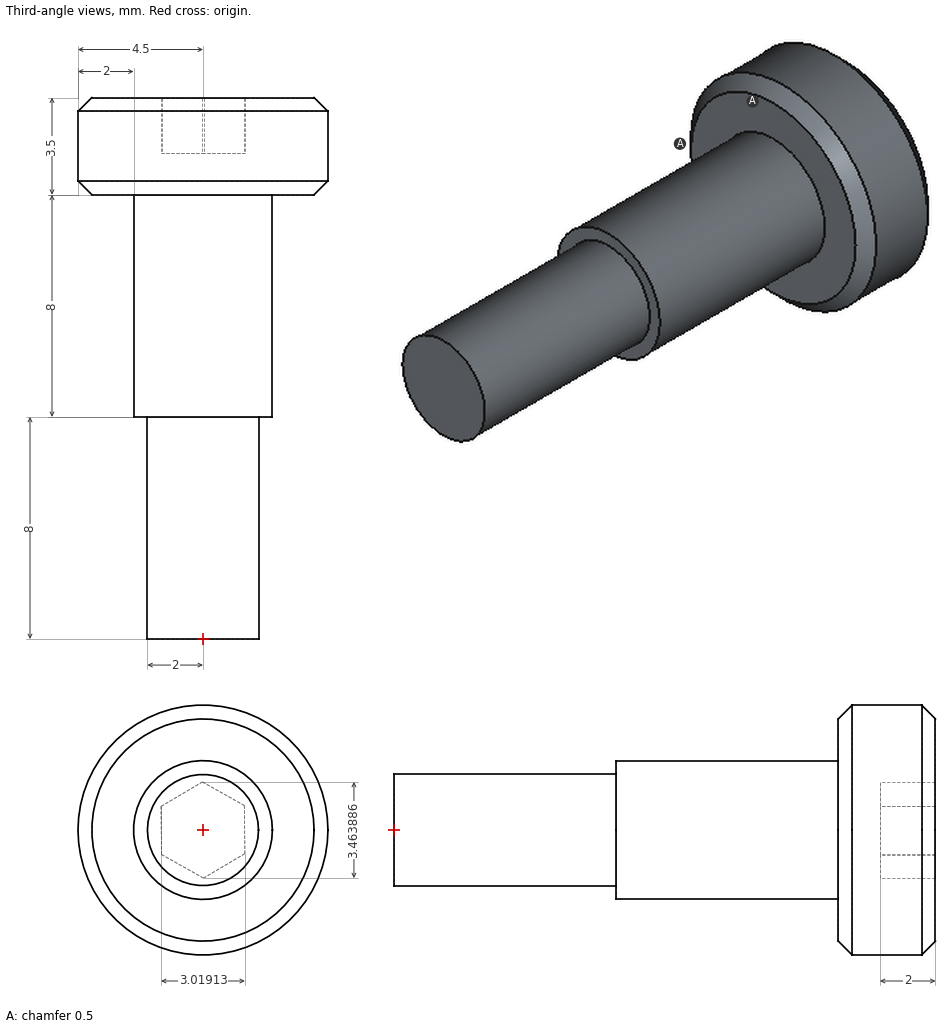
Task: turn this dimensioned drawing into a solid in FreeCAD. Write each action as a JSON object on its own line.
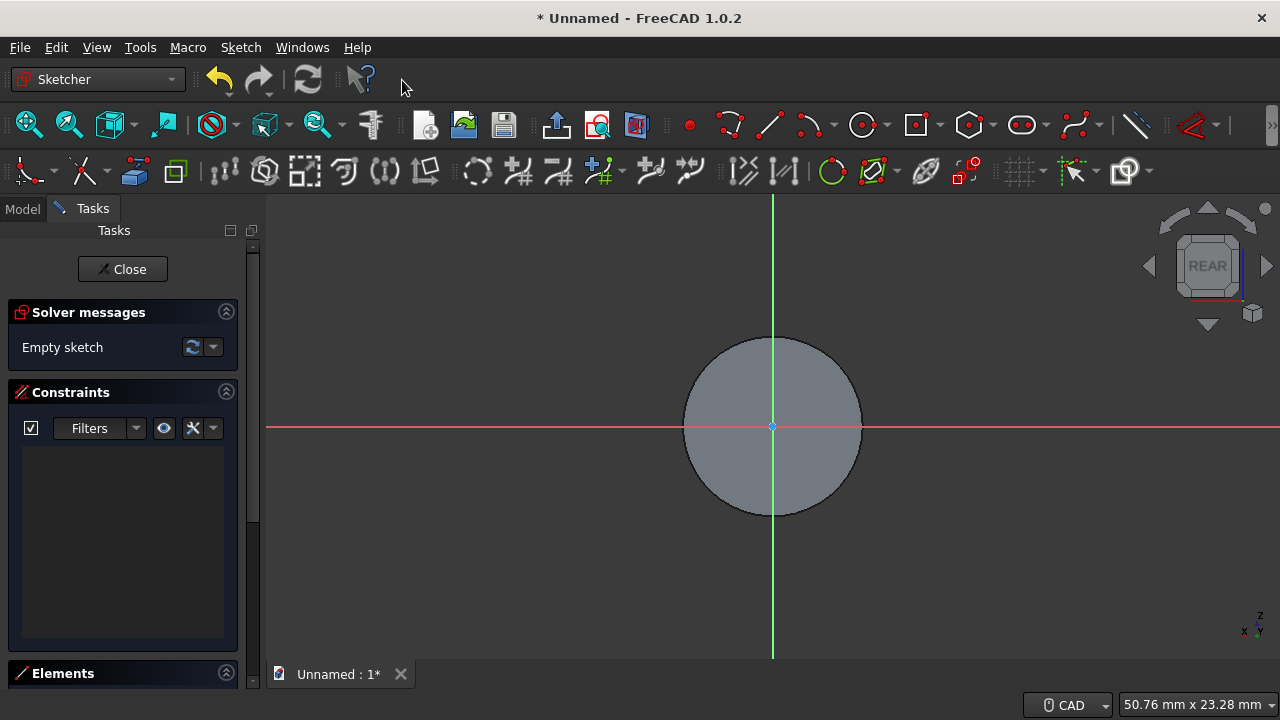
{"action": "scroll", "coordinate": [795, 426], "scroll_direction": "up", "scroll_amount": 7}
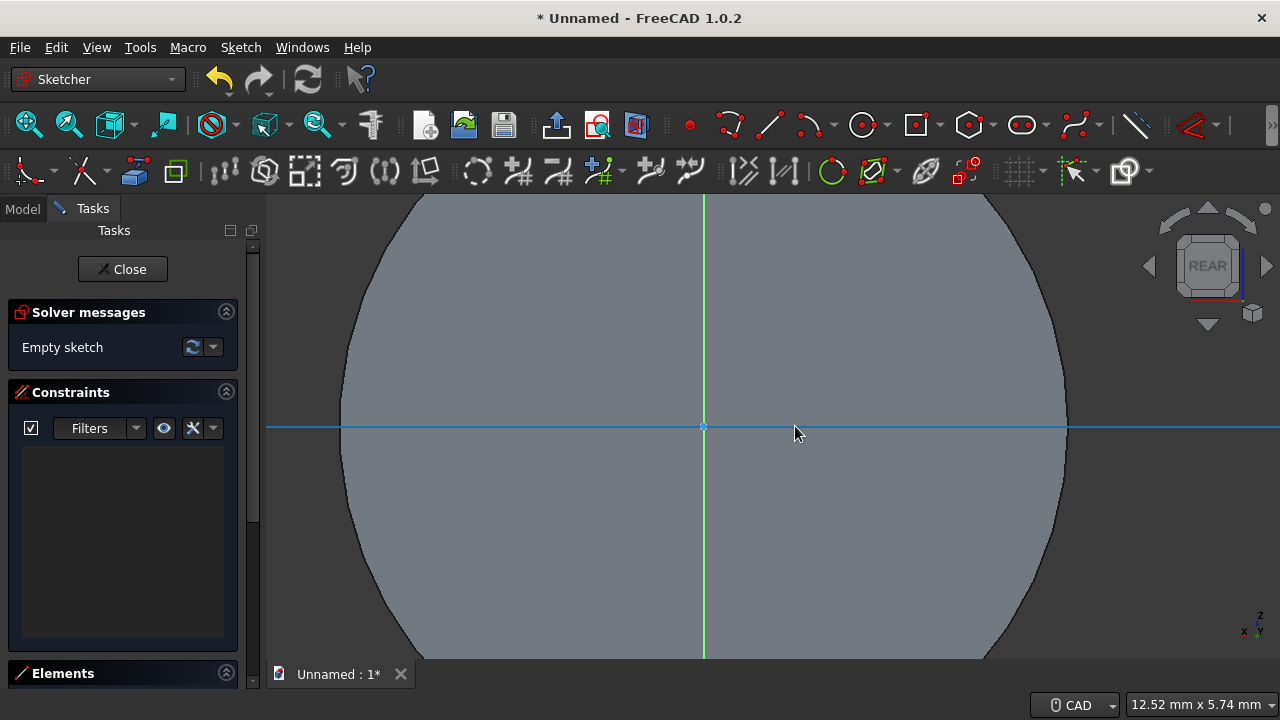
{"action": "left_click", "coordinate": [970, 126]}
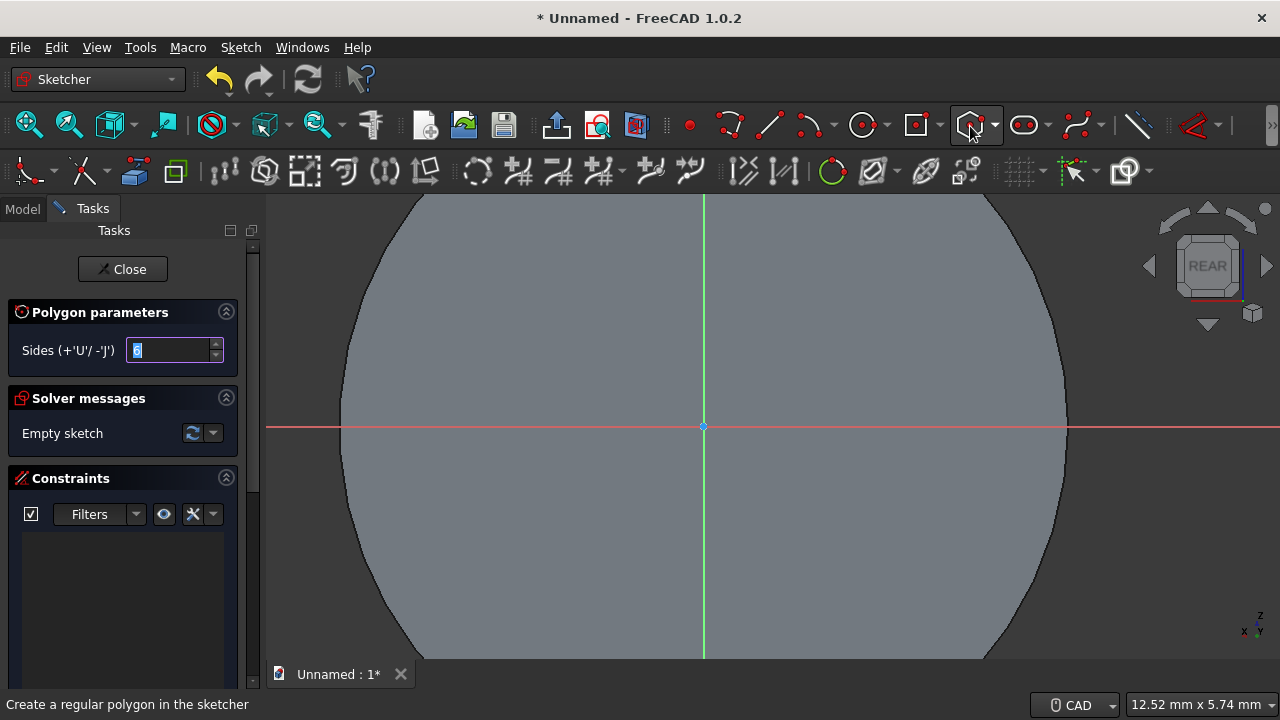
{"action": "left_click", "coordinate": [704, 426]}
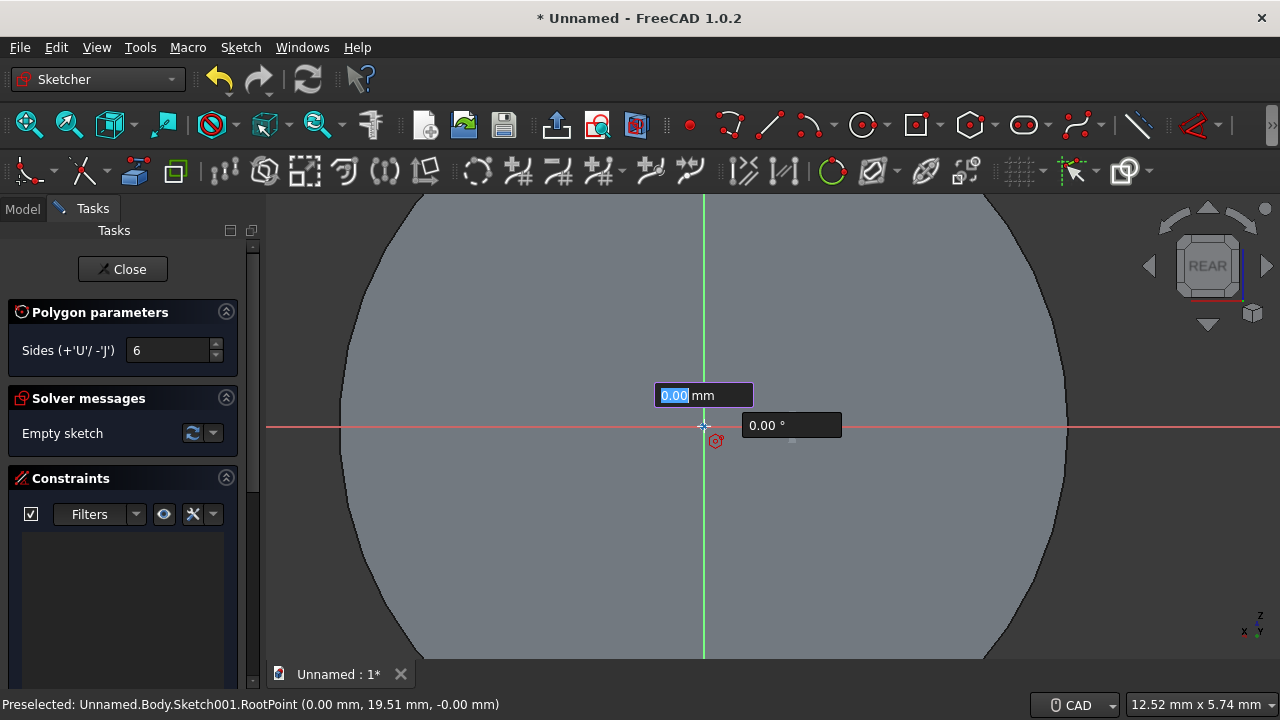
{"action": "left_click", "coordinate": [824, 498]}
{"action": "right_click", "coordinate": [824, 498]}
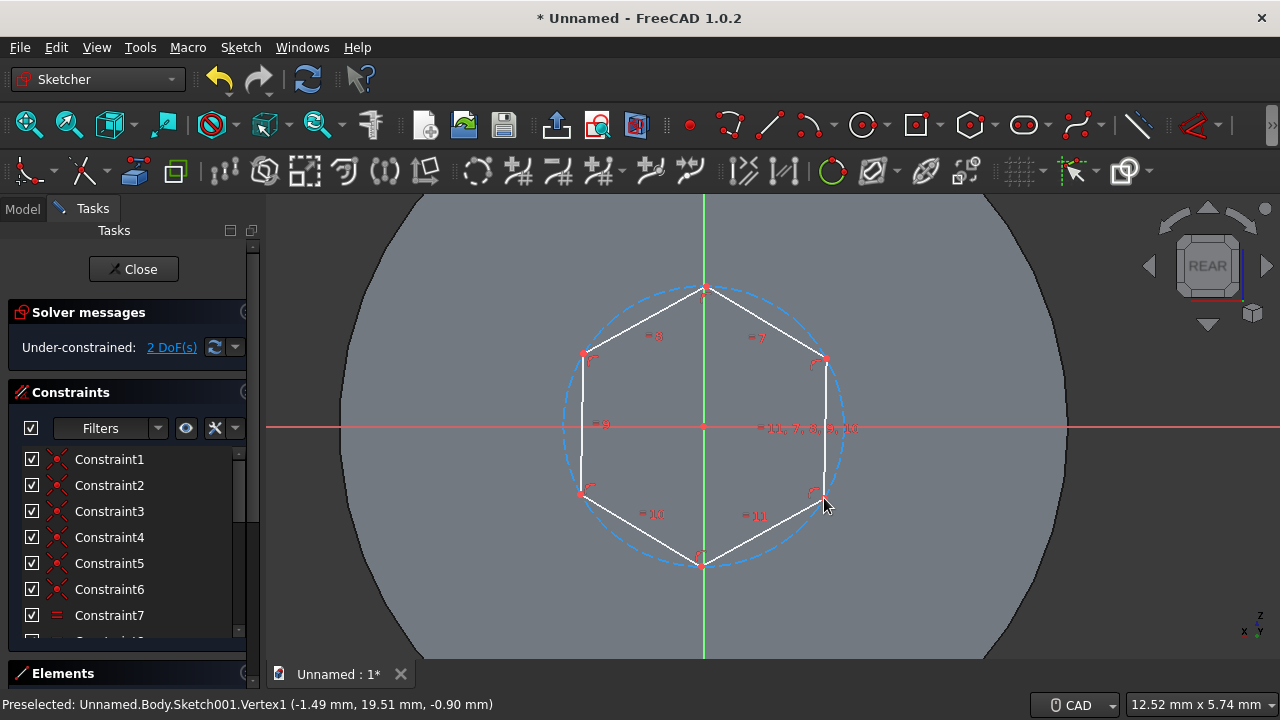
{"action": "key", "text": "d"}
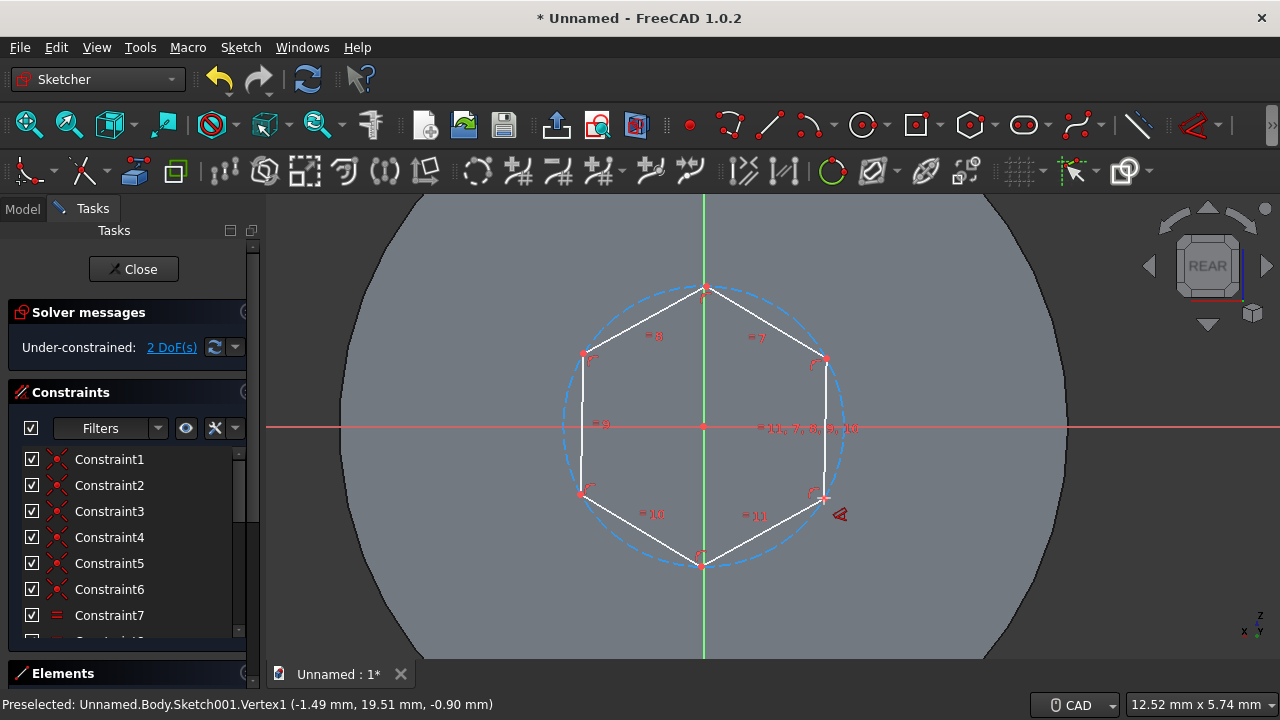
{"action": "left_click", "coordinate": [581, 494]}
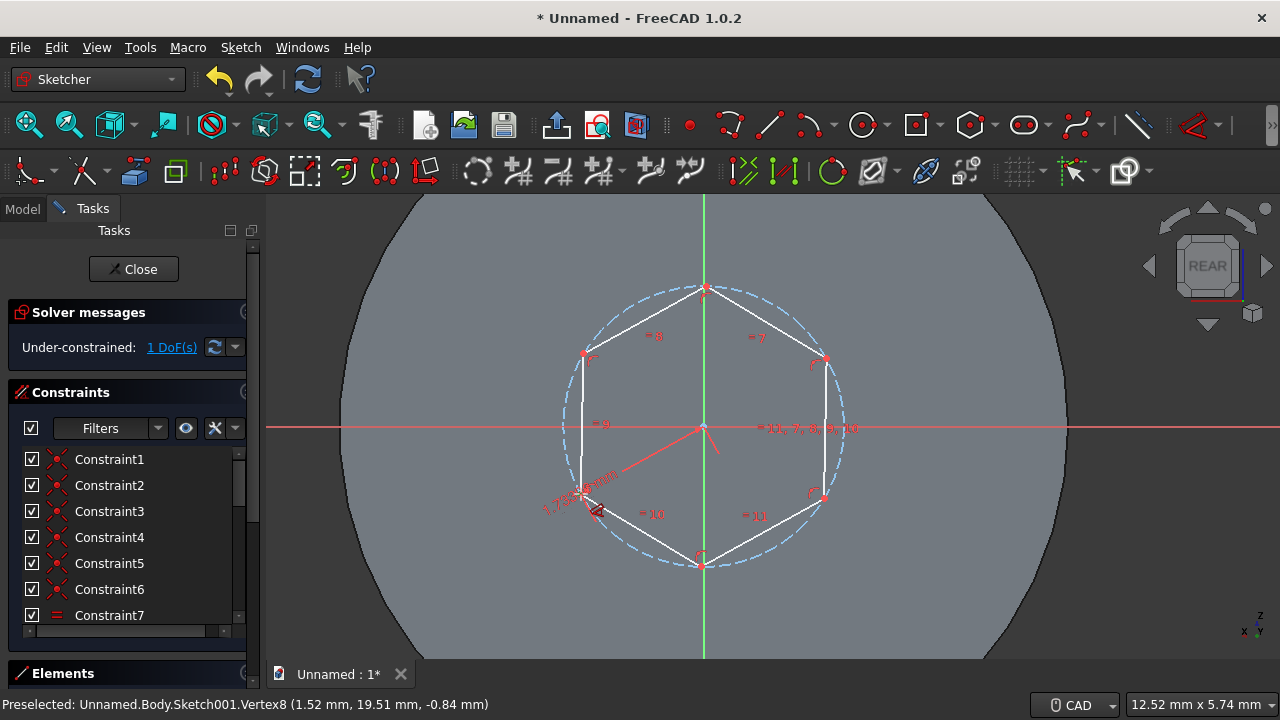
{"action": "left_click", "coordinate": [827, 359]}
{"action": "left_click", "coordinate": [647, 576]}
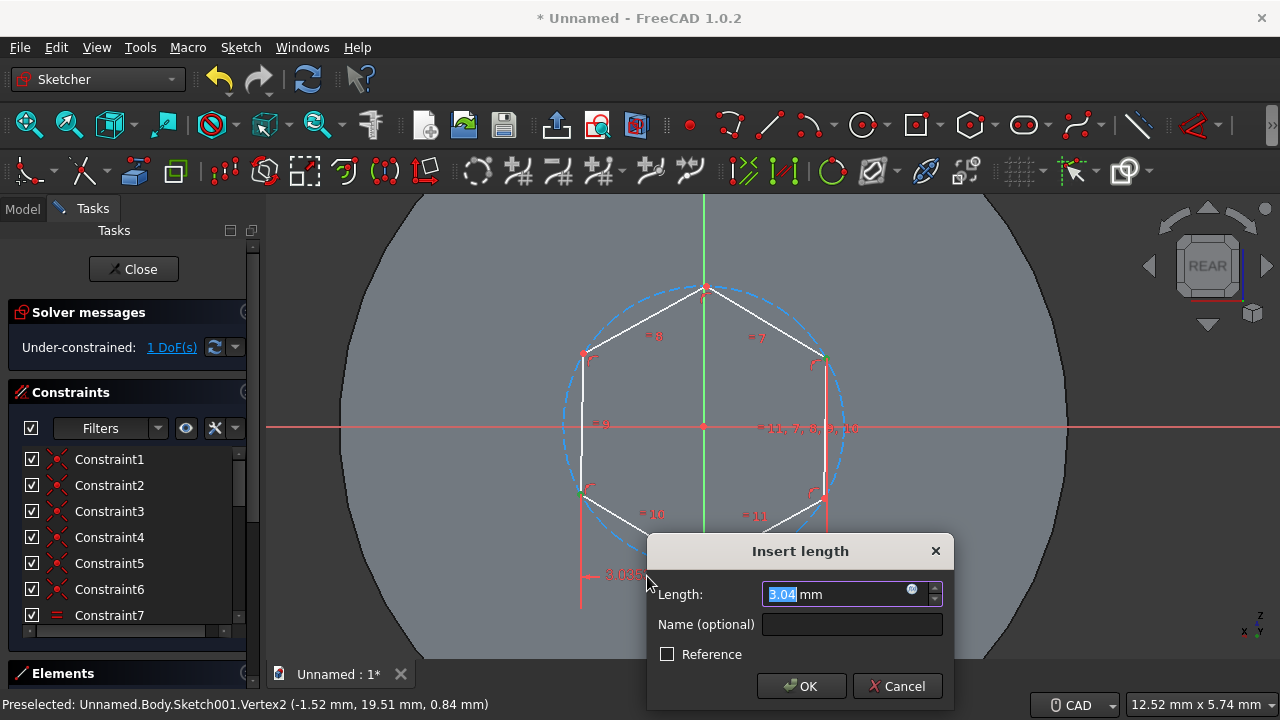
{"action": "type", "text": "3.01913"}
{"action": "key", "text": "Return"}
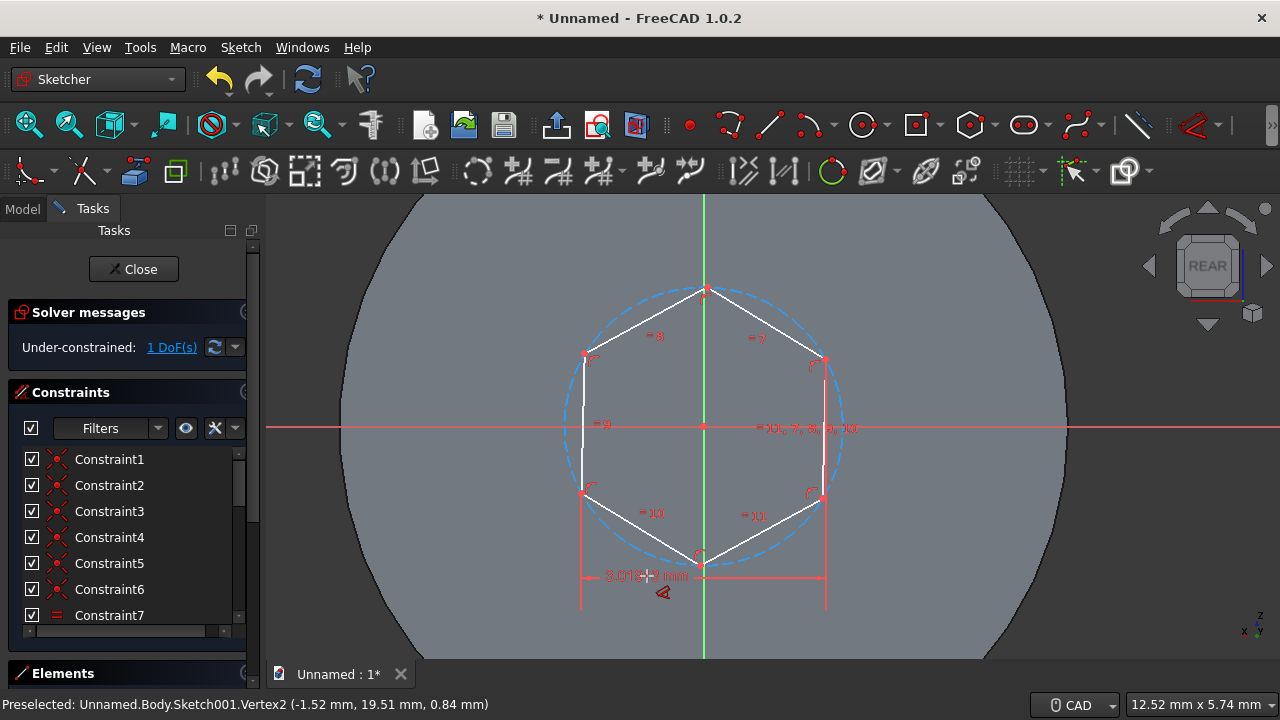
{"action": "left_click", "coordinate": [700, 566]}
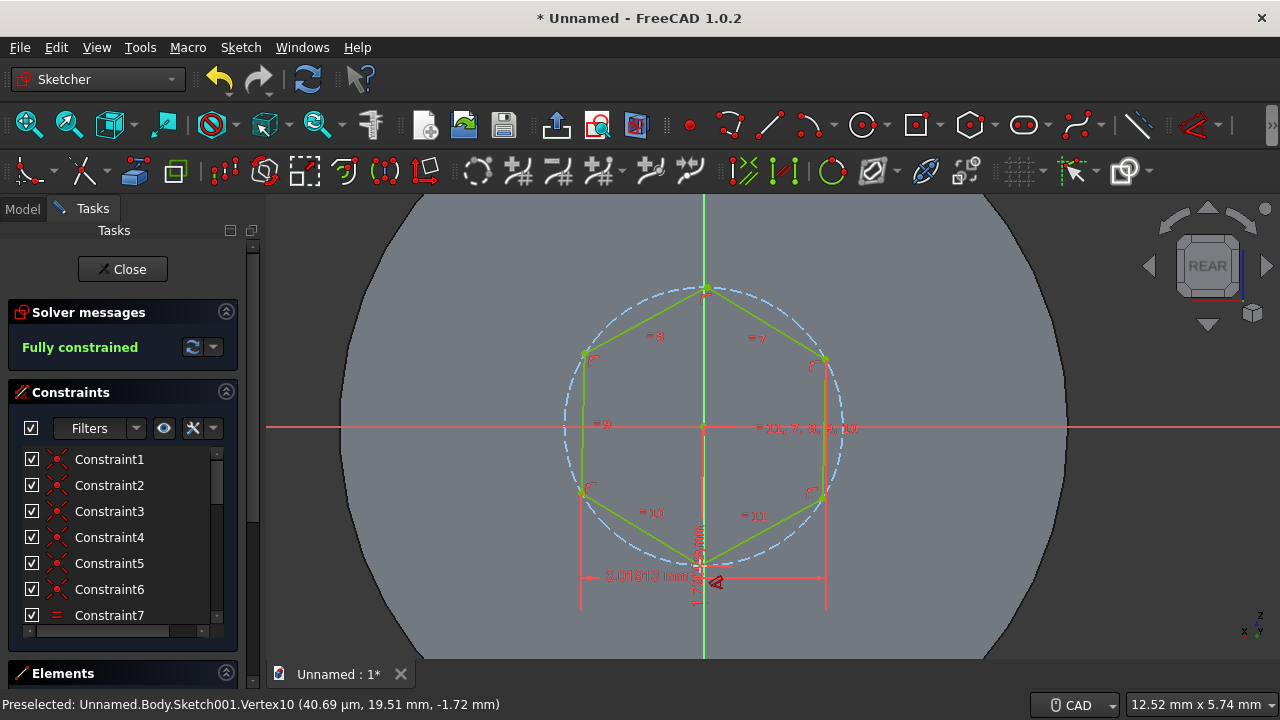
{"action": "left_click", "coordinate": [707, 287]}
{"action": "left_click", "coordinate": [741, 362]}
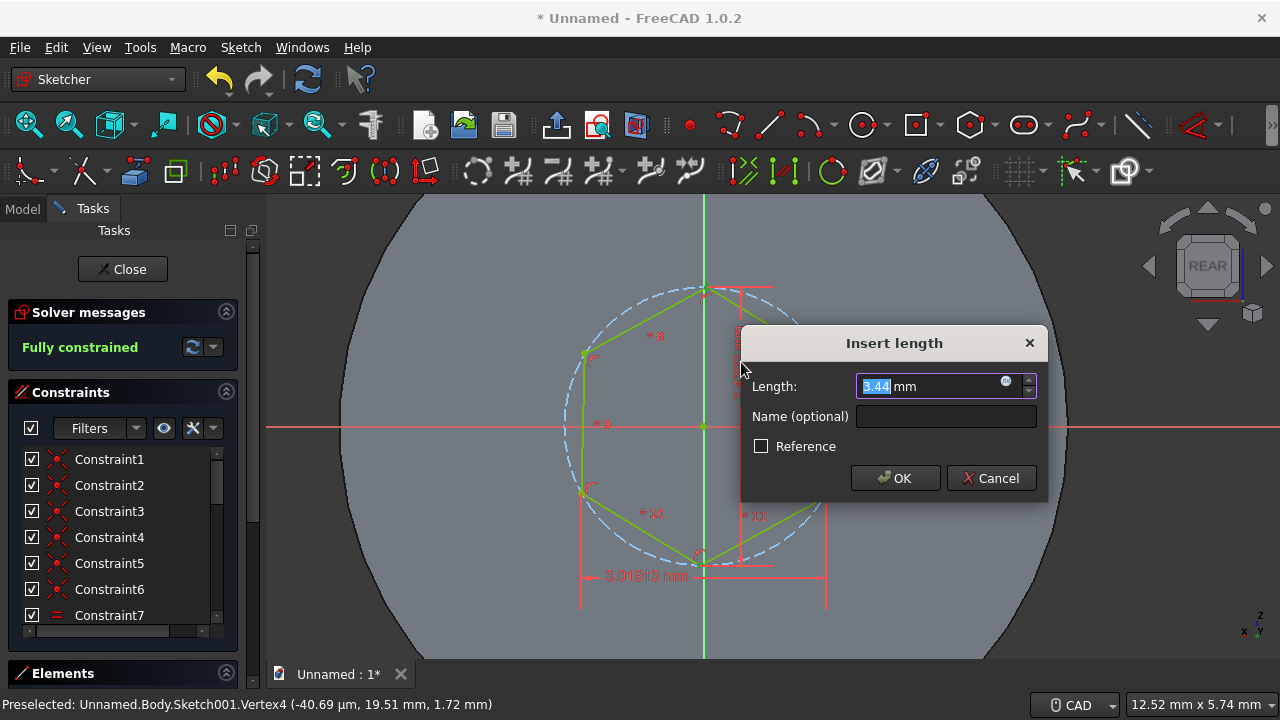
{"action": "type", "text": "3.463886"}
{"action": "key", "text": "Return"}
{"action": "key", "text": "Escape"}